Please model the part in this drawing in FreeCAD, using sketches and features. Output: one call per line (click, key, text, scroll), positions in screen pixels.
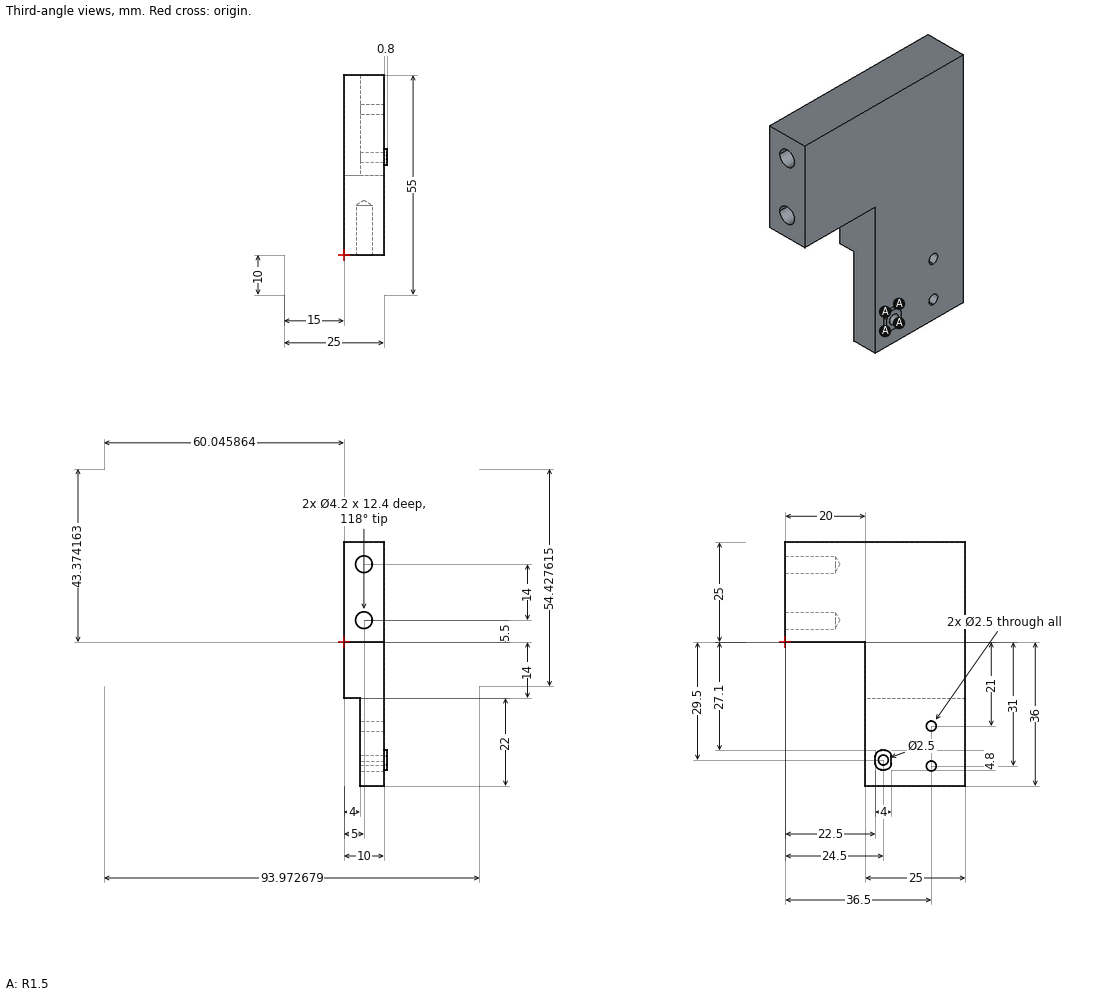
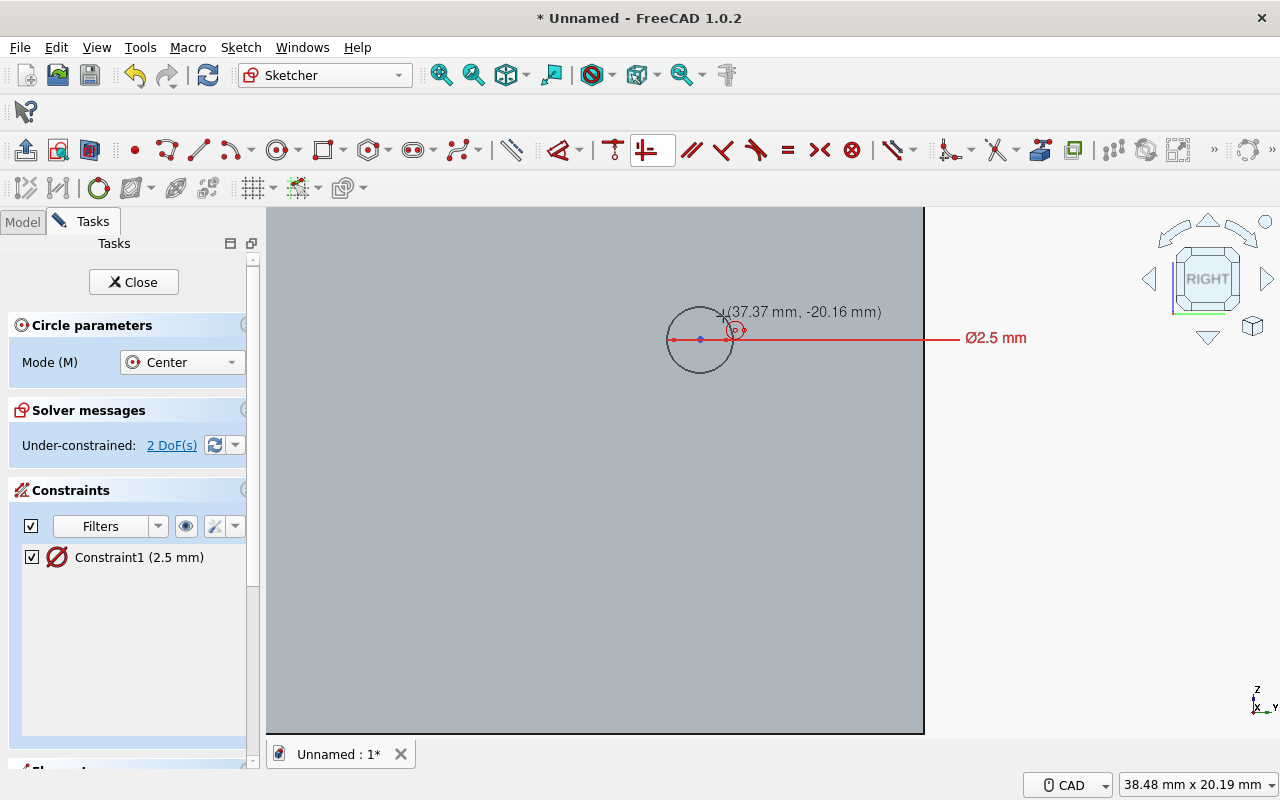
click(700, 603)
move(723, 579)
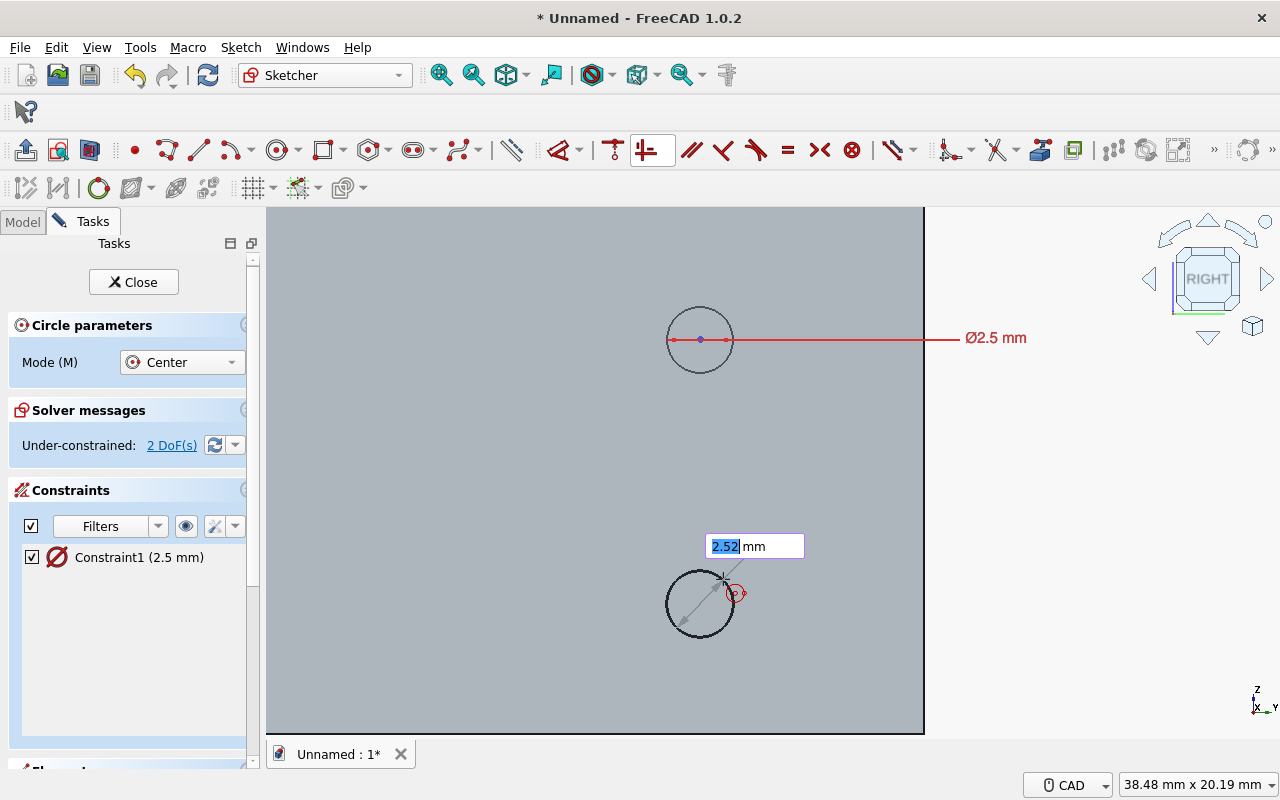
text(2.5)
key(Return)
key(Escape)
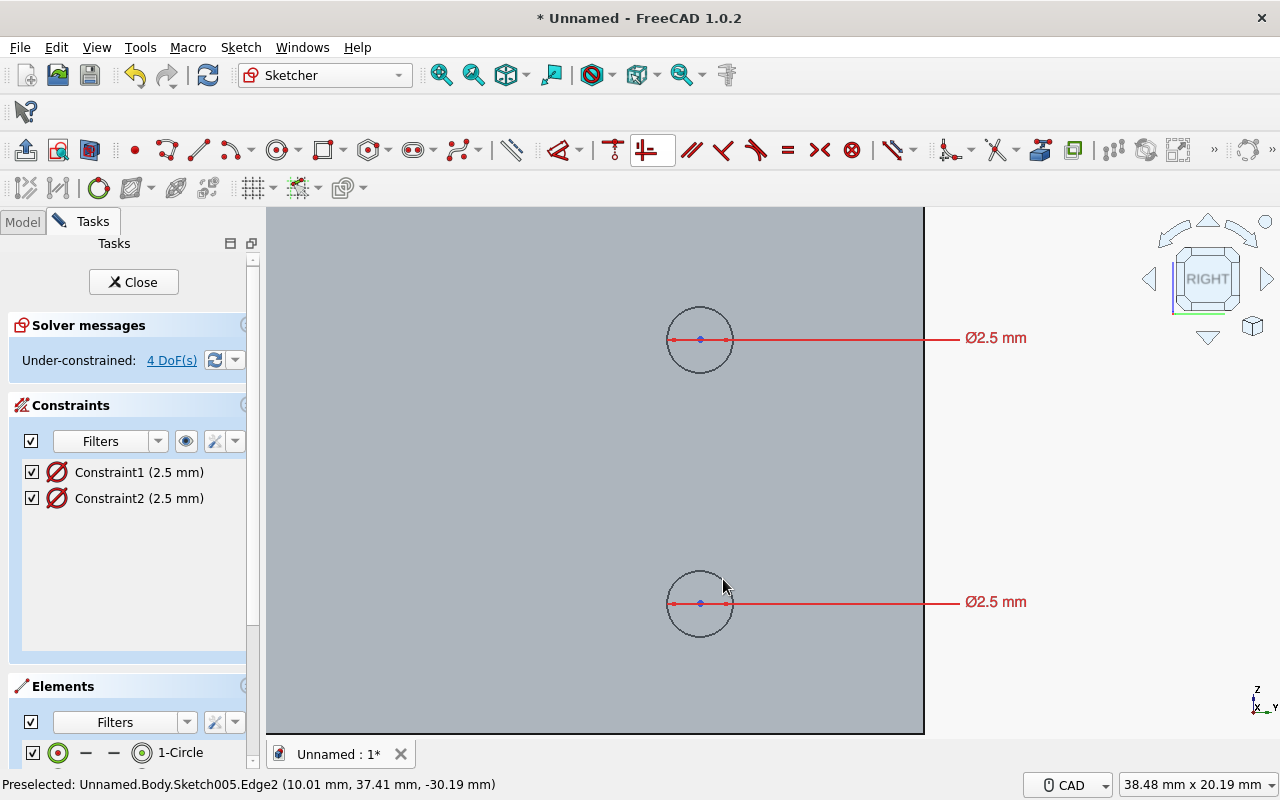
click(700, 340)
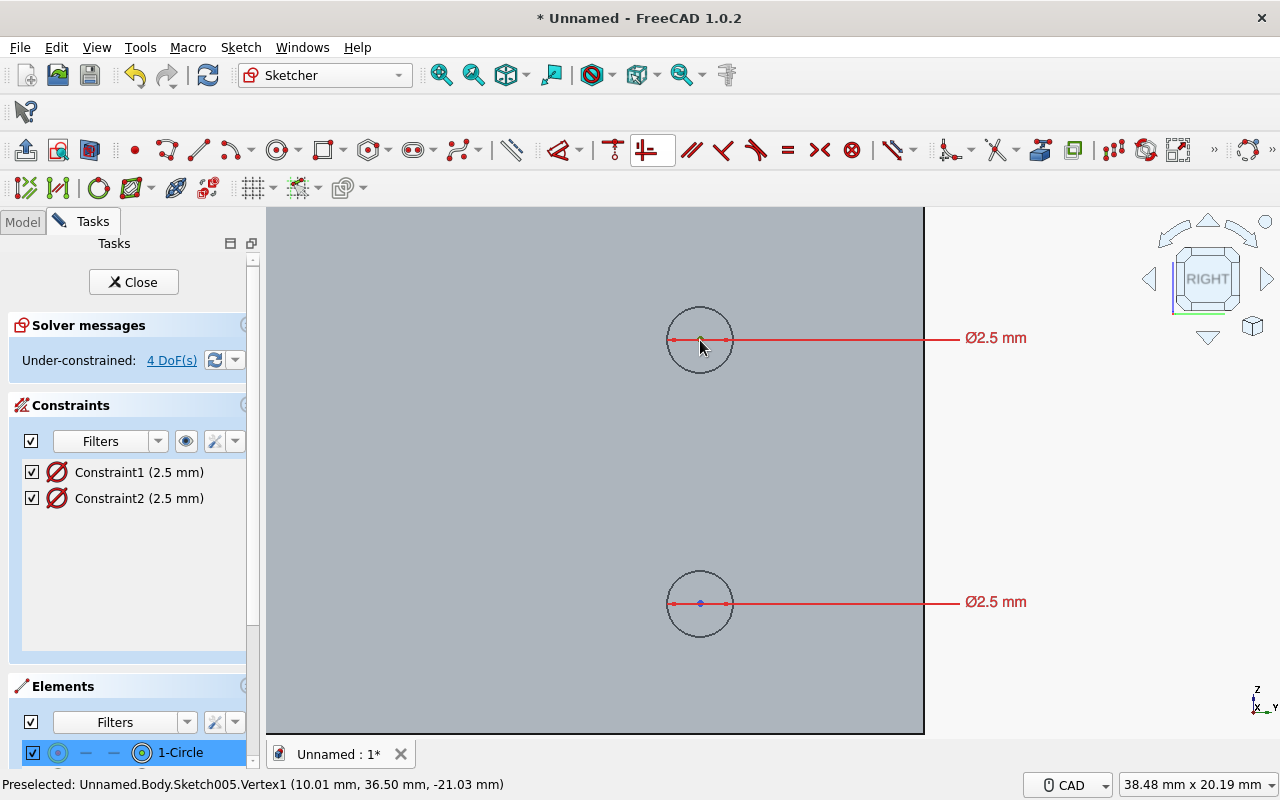
click(700, 604)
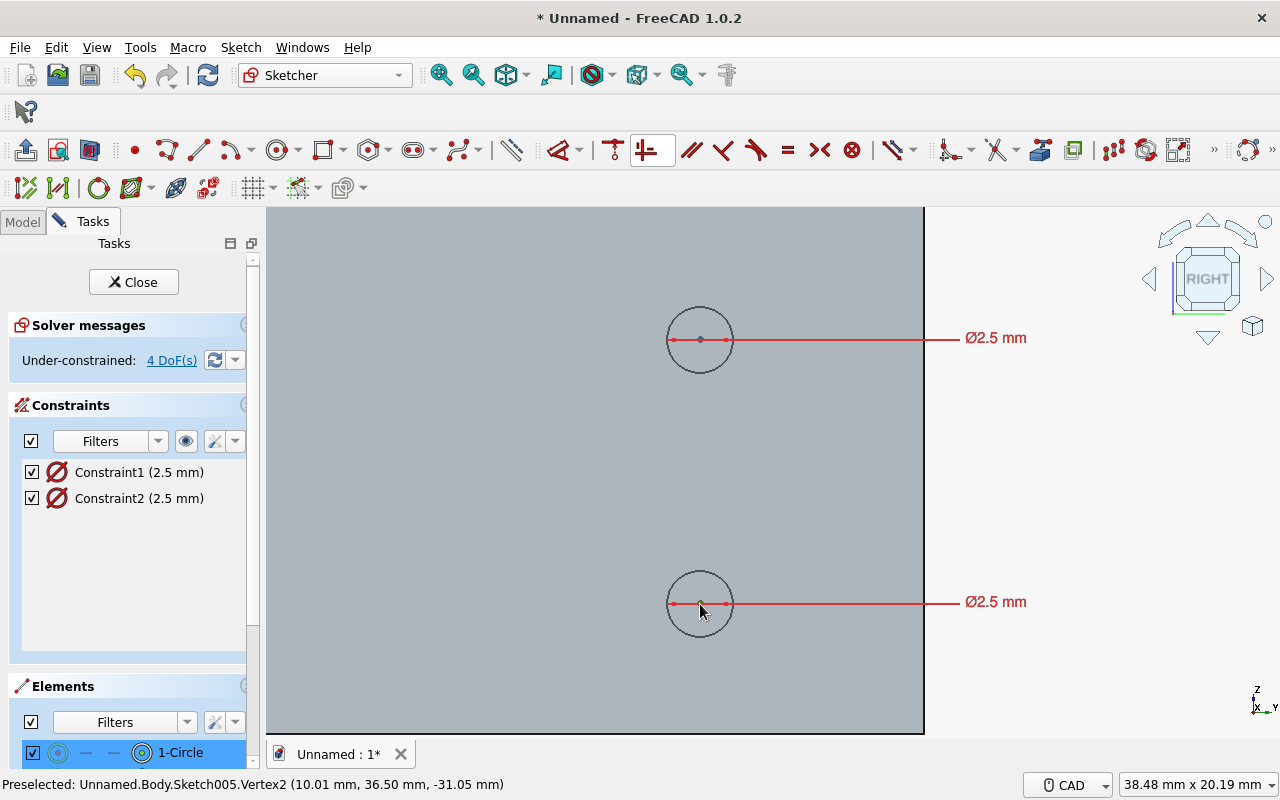
click(670, 150)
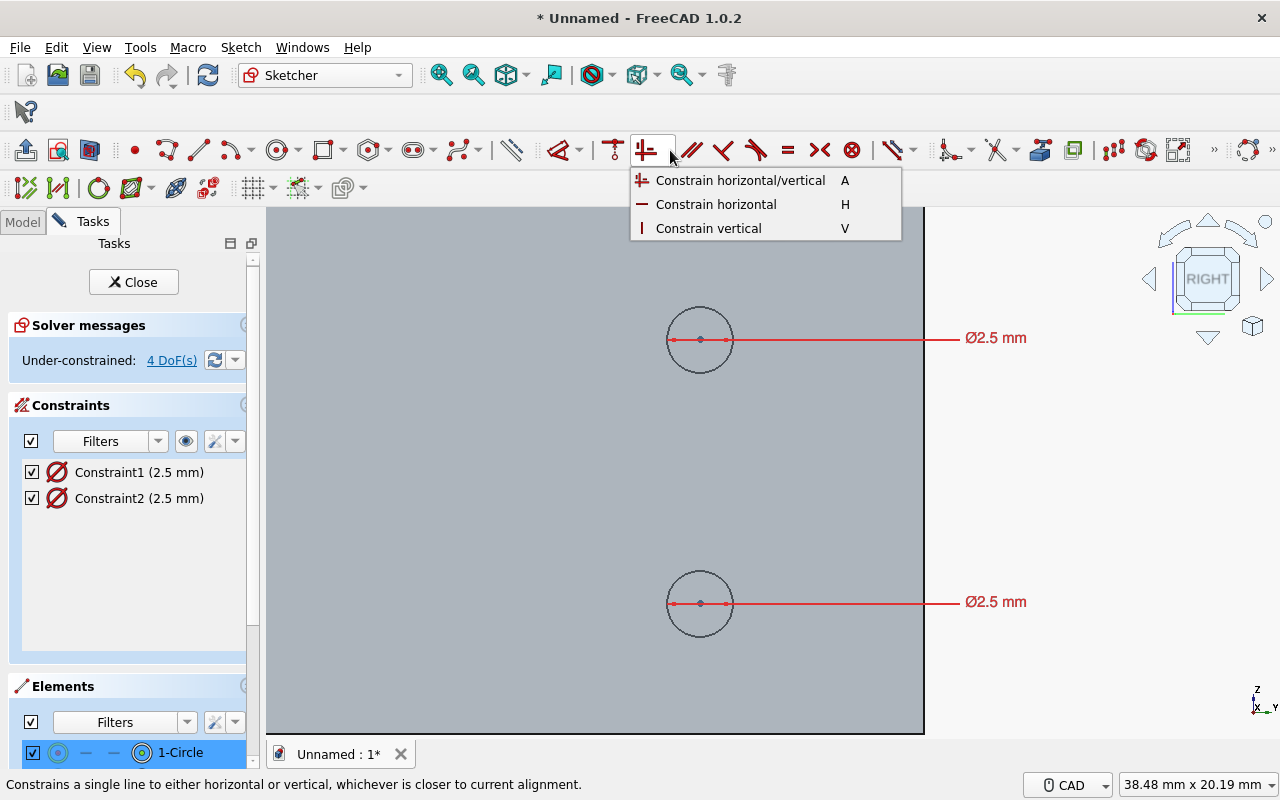
click(766, 228)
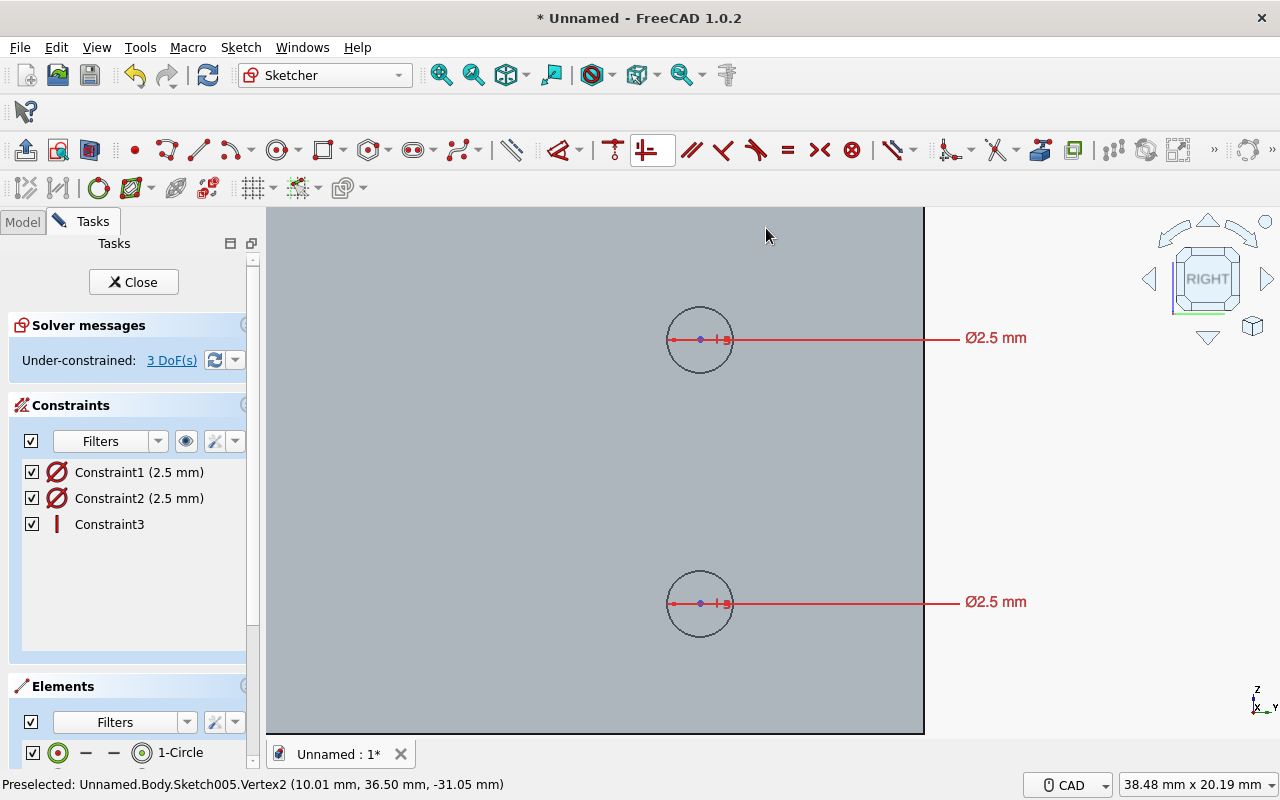
click(558, 150)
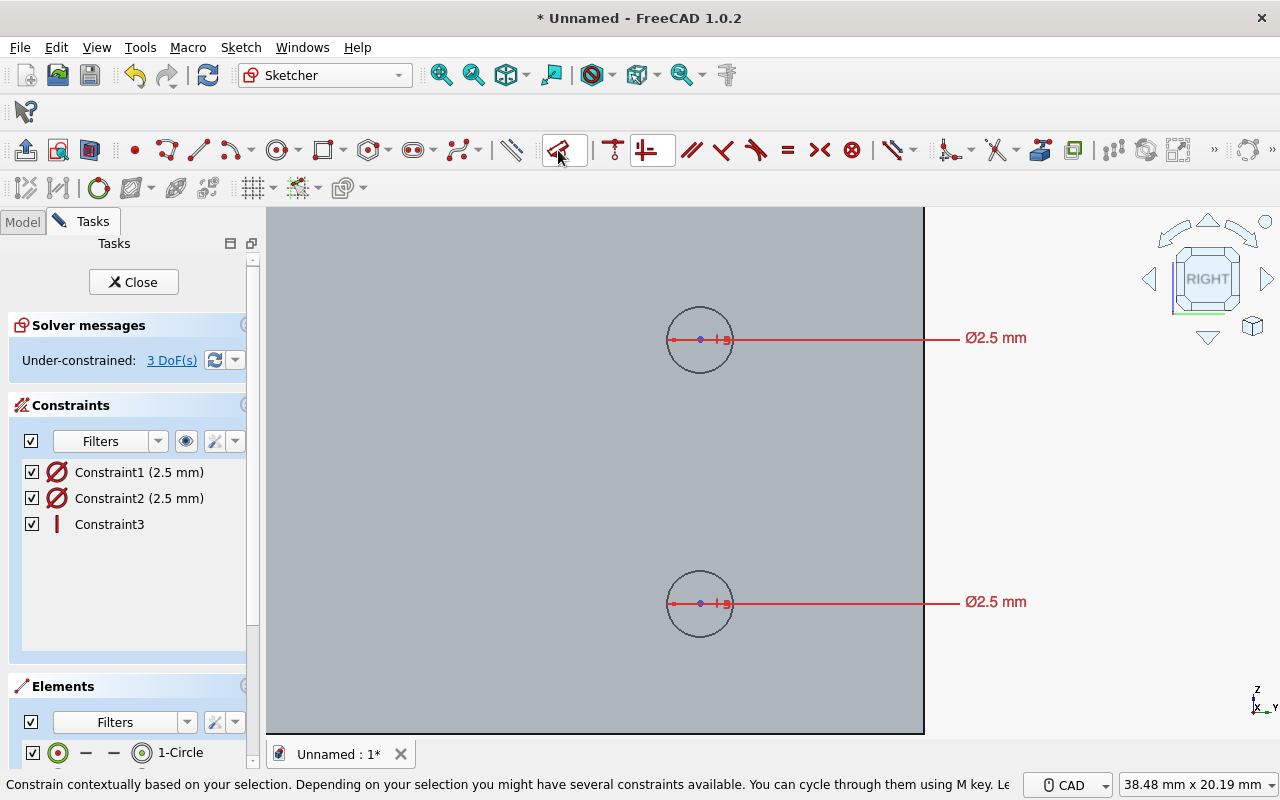
click(700, 340)
click(734, 288)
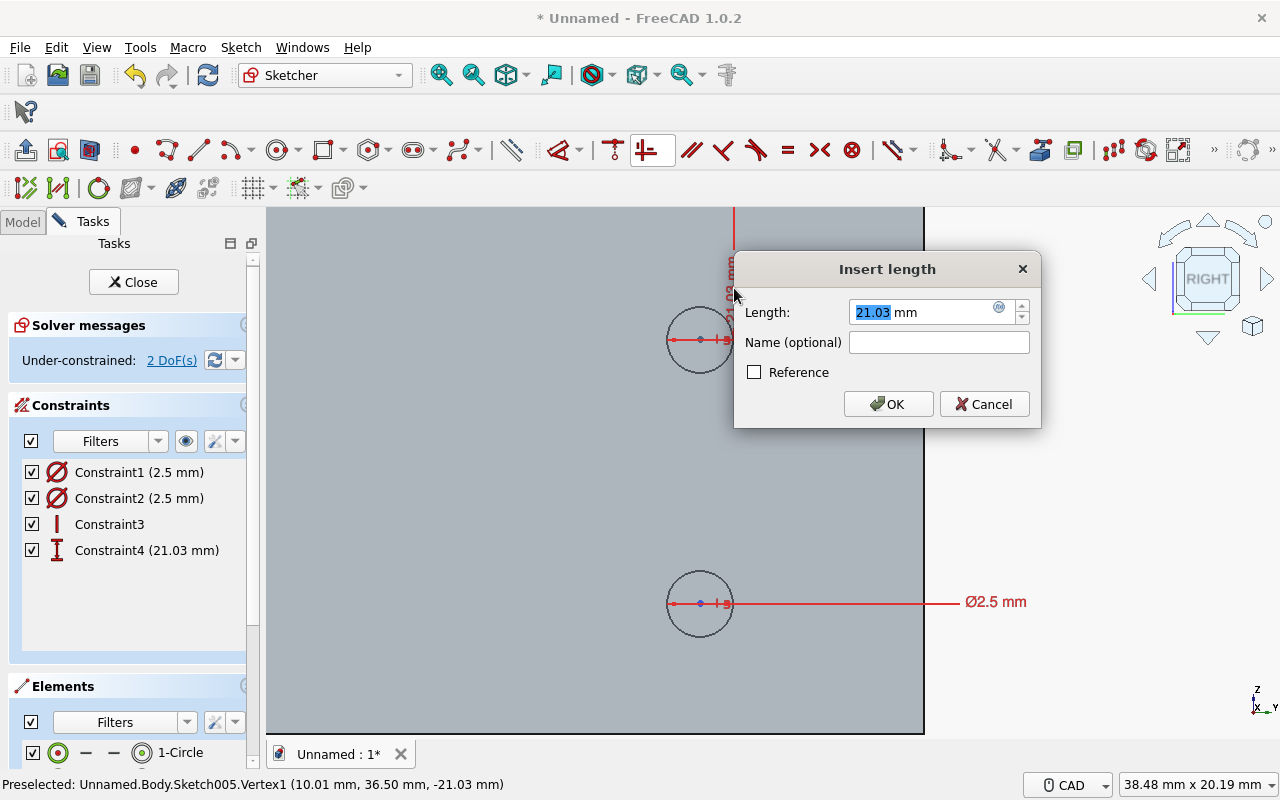
text(21)
key(Return)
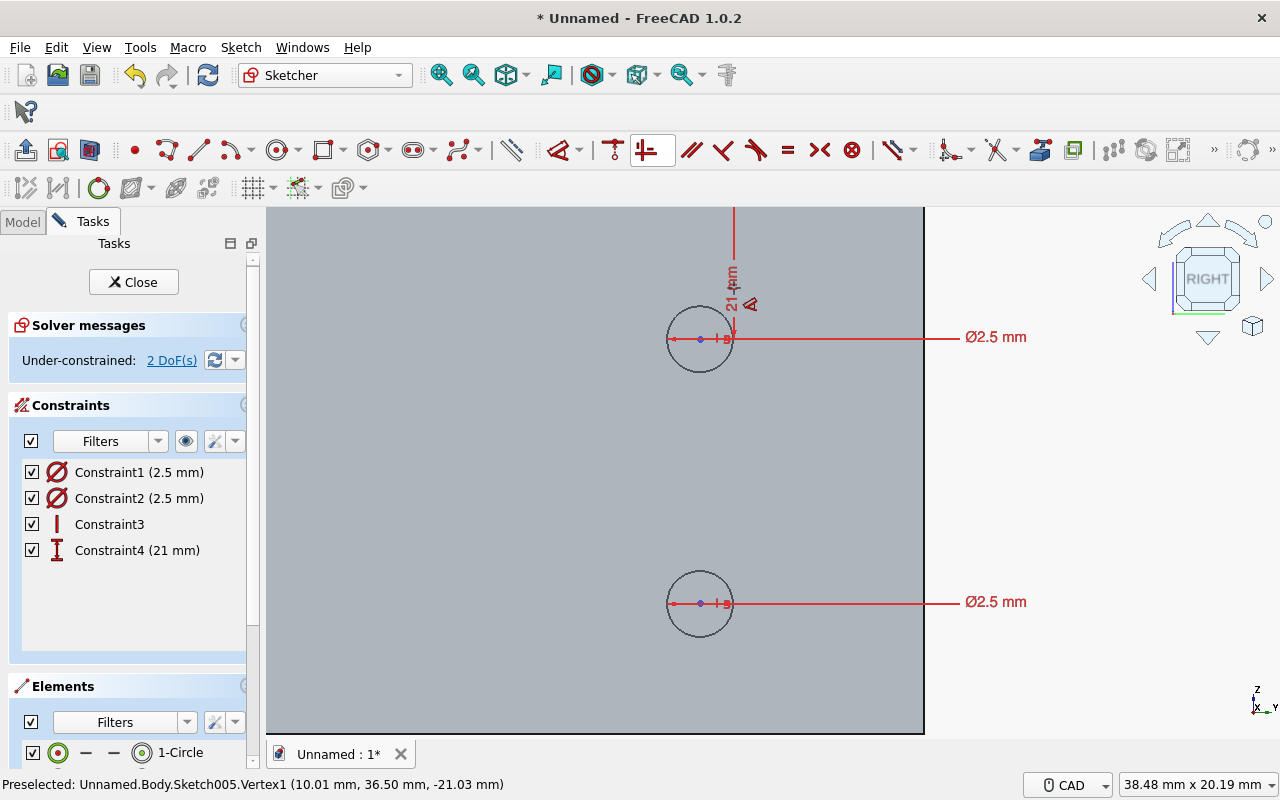
click(700, 604)
click(734, 420)